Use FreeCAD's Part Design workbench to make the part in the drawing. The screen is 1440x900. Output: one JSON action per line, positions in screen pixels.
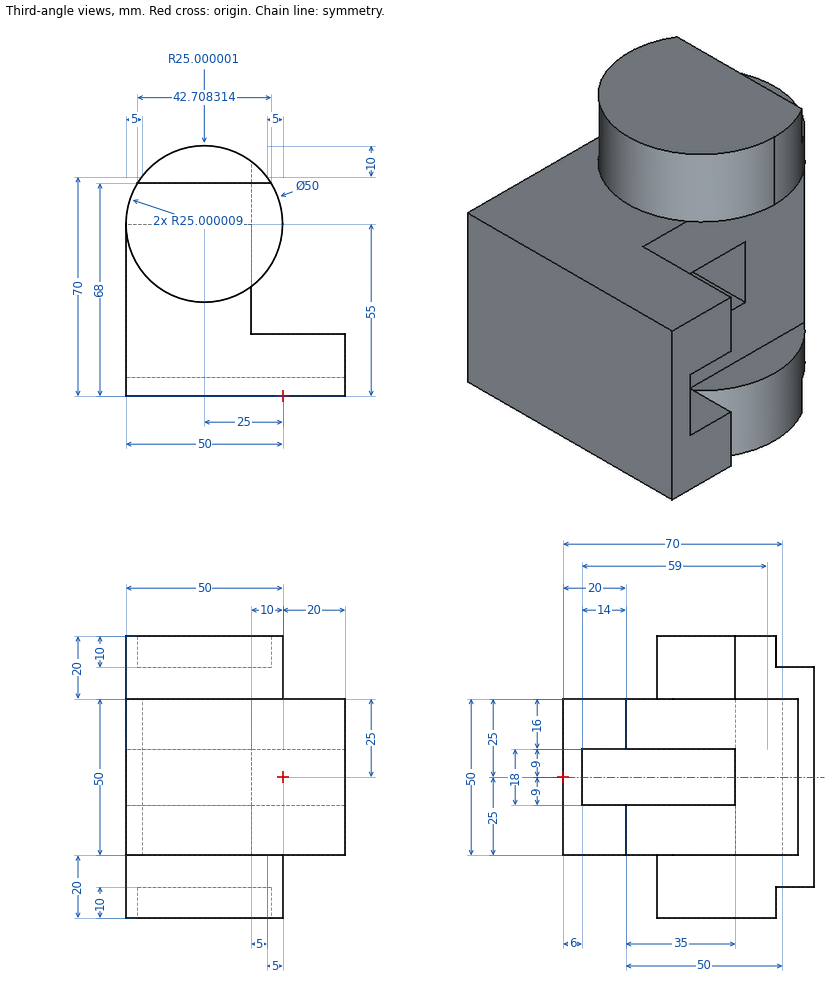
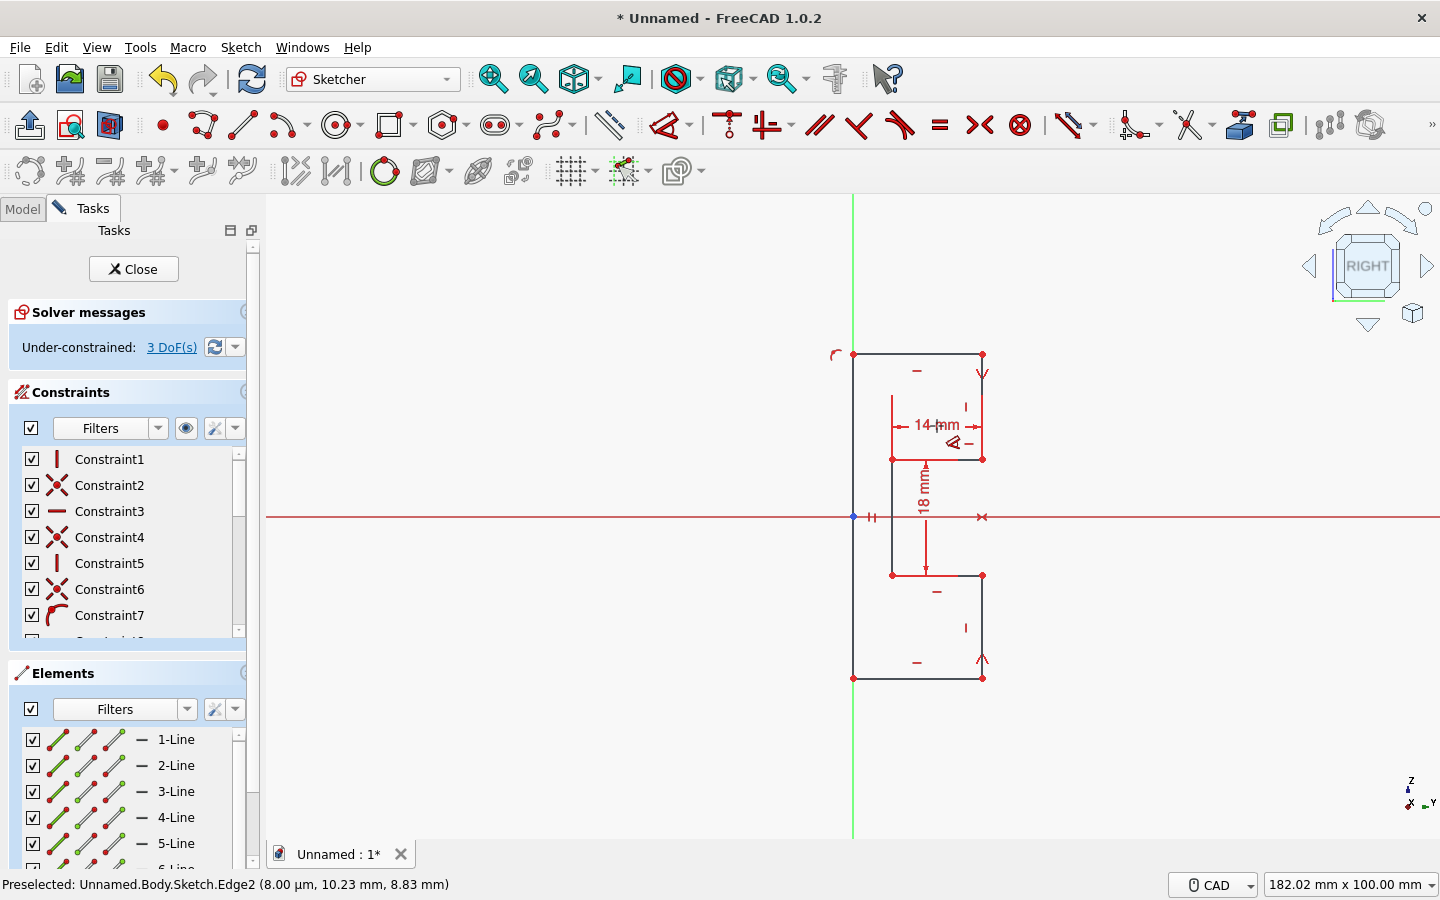
{"action": "left_click", "coordinate": [982, 428]}
{"action": "left_click", "coordinate": [1016, 407]}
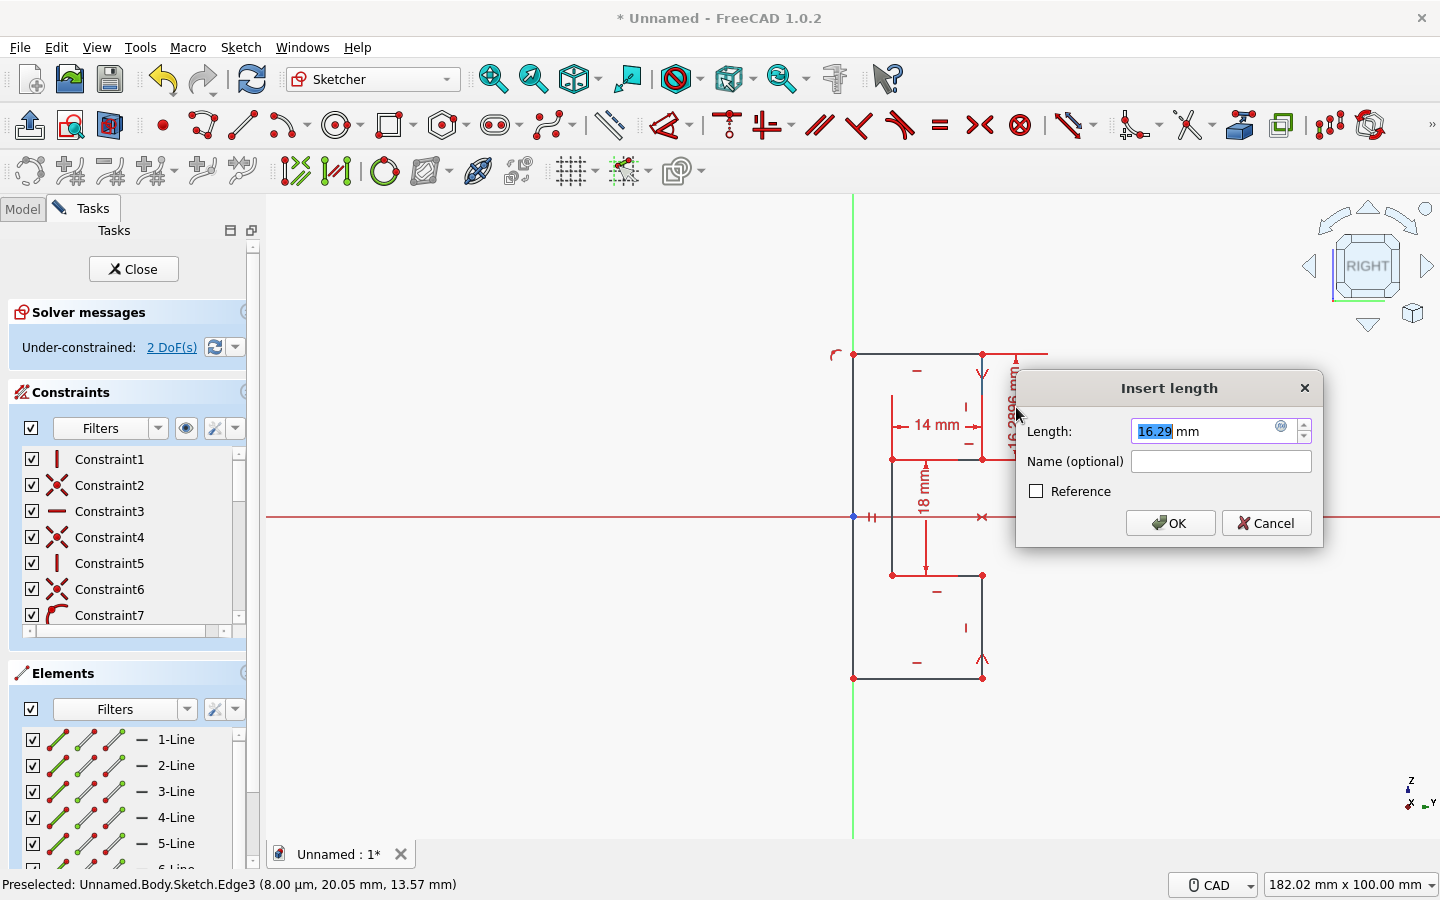
{"action": "type", "text": "16"}
{"action": "key", "text": "Return"}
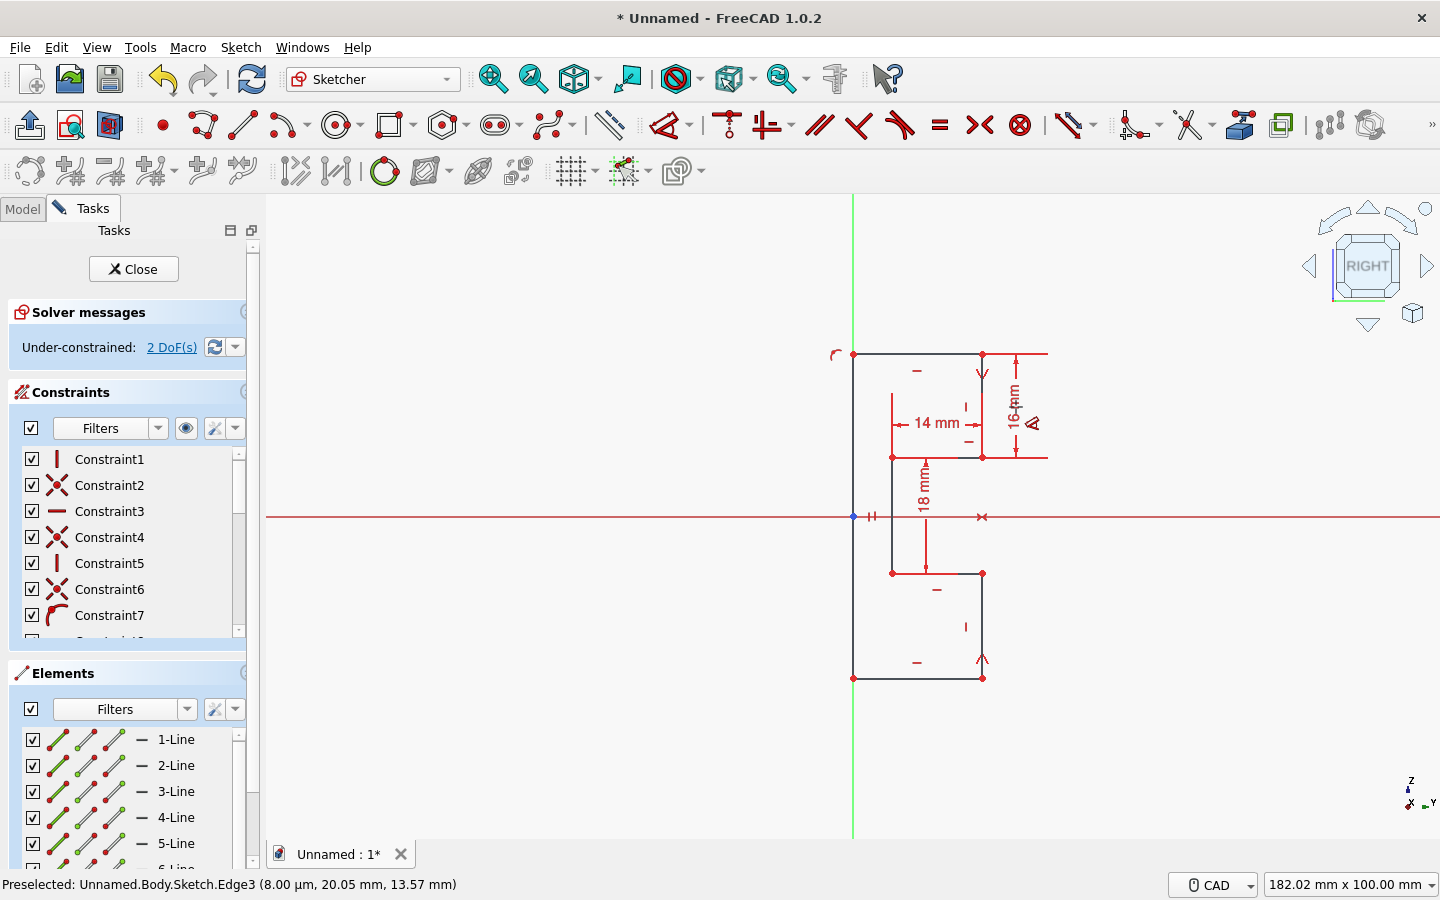
{"action": "left_click", "coordinate": [944, 354]}
{"action": "left_click", "coordinate": [918, 320]}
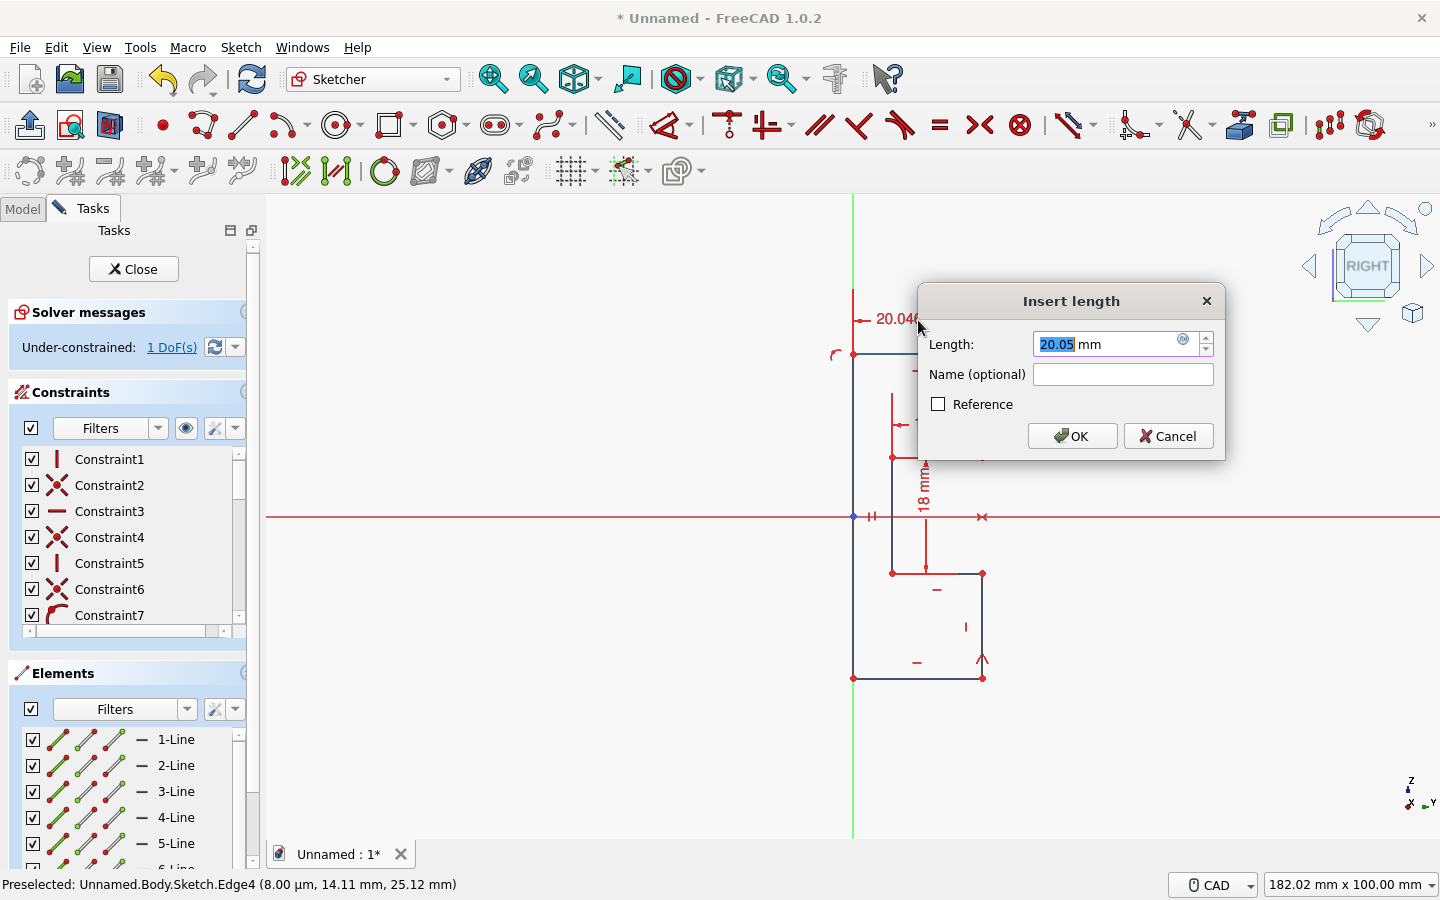
{"action": "type", "text": "20"}
{"action": "key", "text": "Return"}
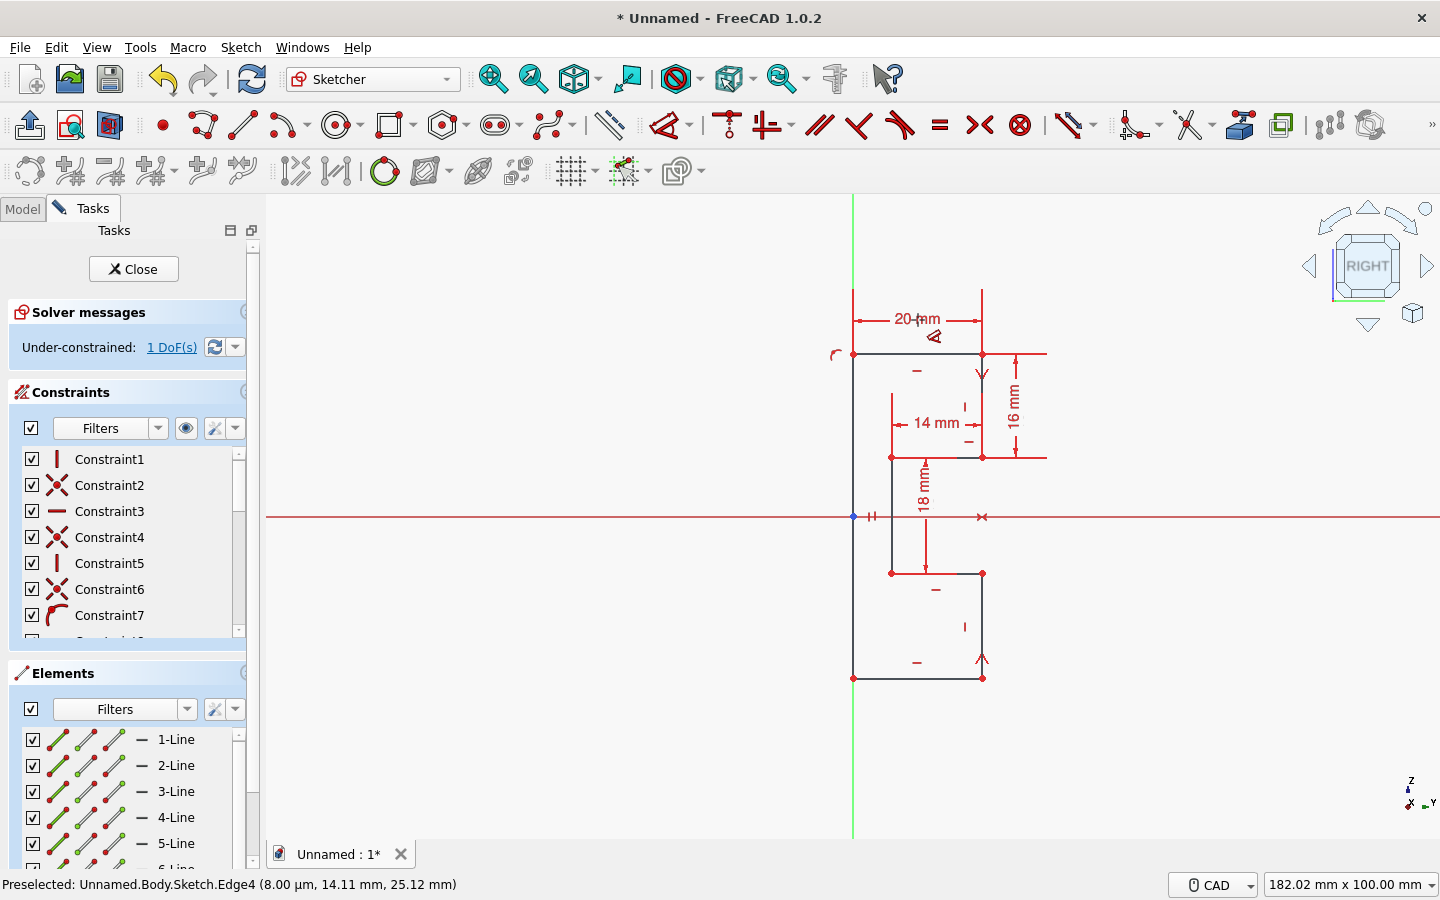
{"action": "left_click", "coordinate": [853, 452]}
{"action": "left_click", "coordinate": [819, 442]}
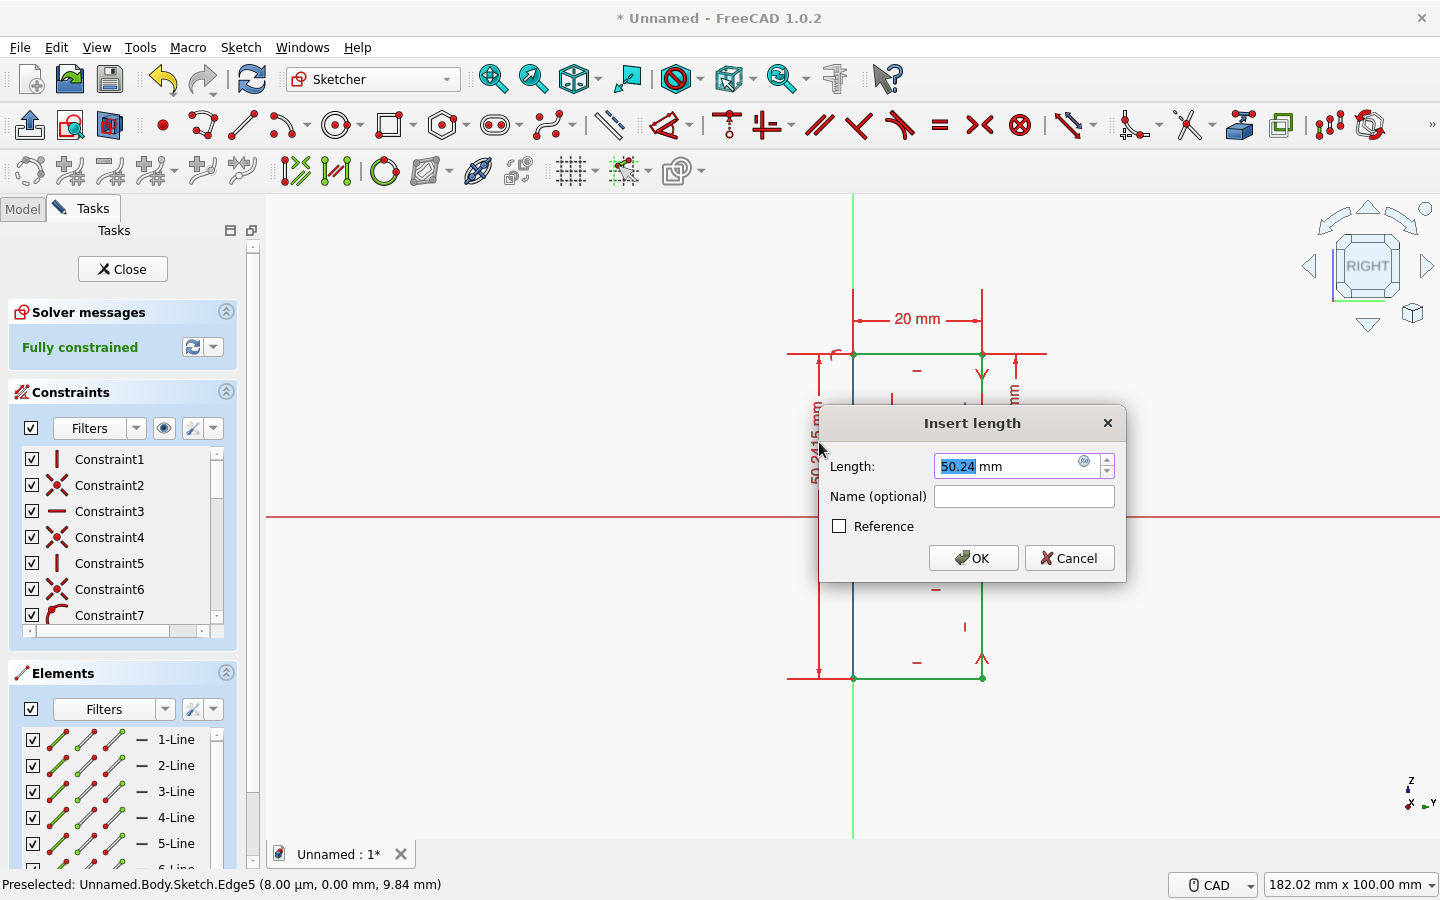
{"action": "type", "text": "50"}
{"action": "key", "text": "Return"}
{"action": "key", "text": "Escape"}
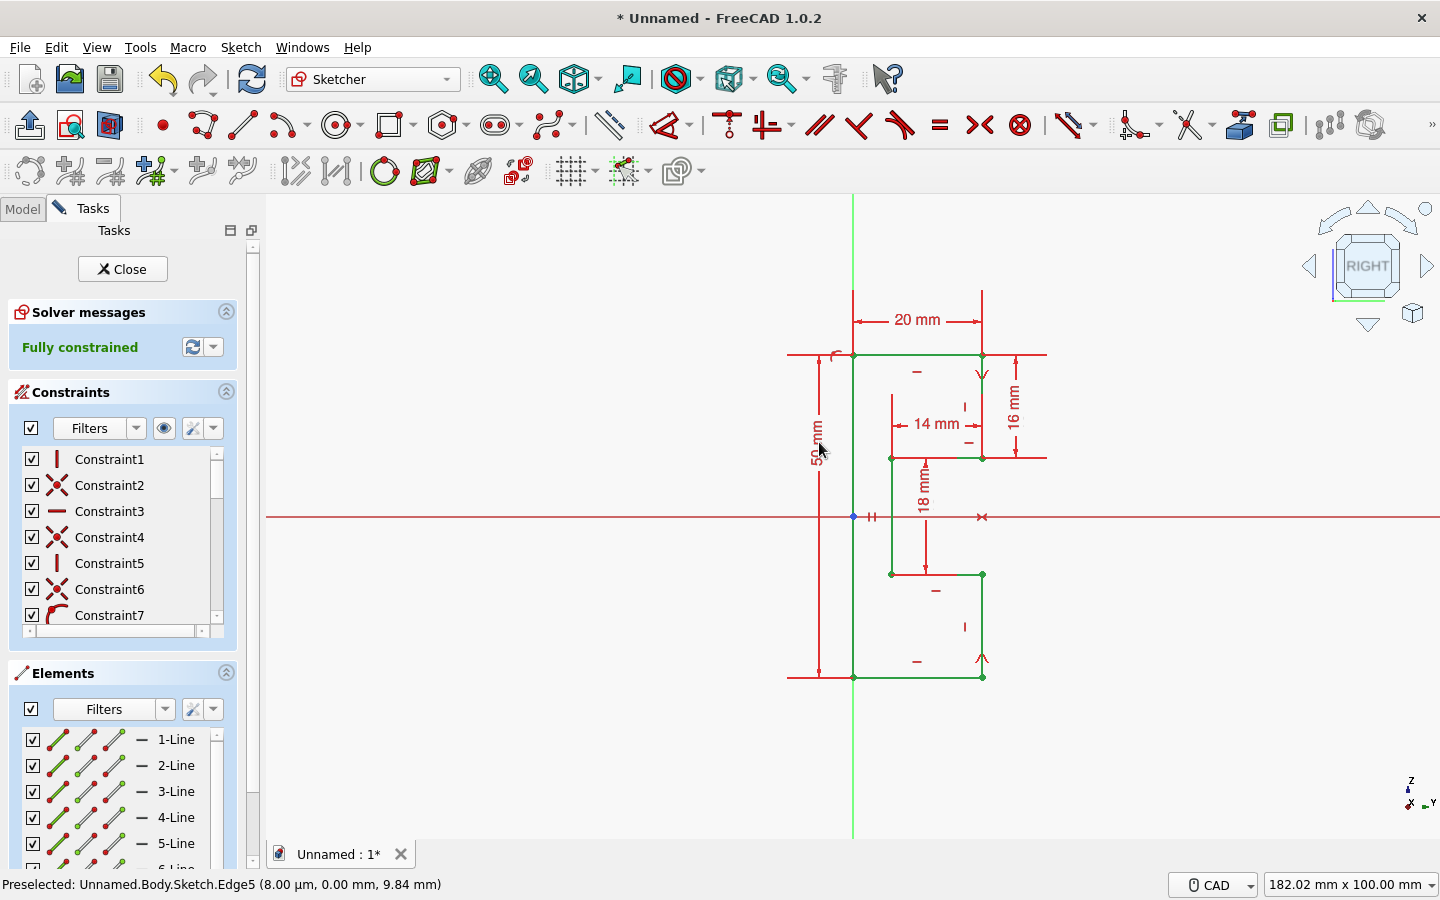
{"action": "left_click", "coordinate": [123, 269]}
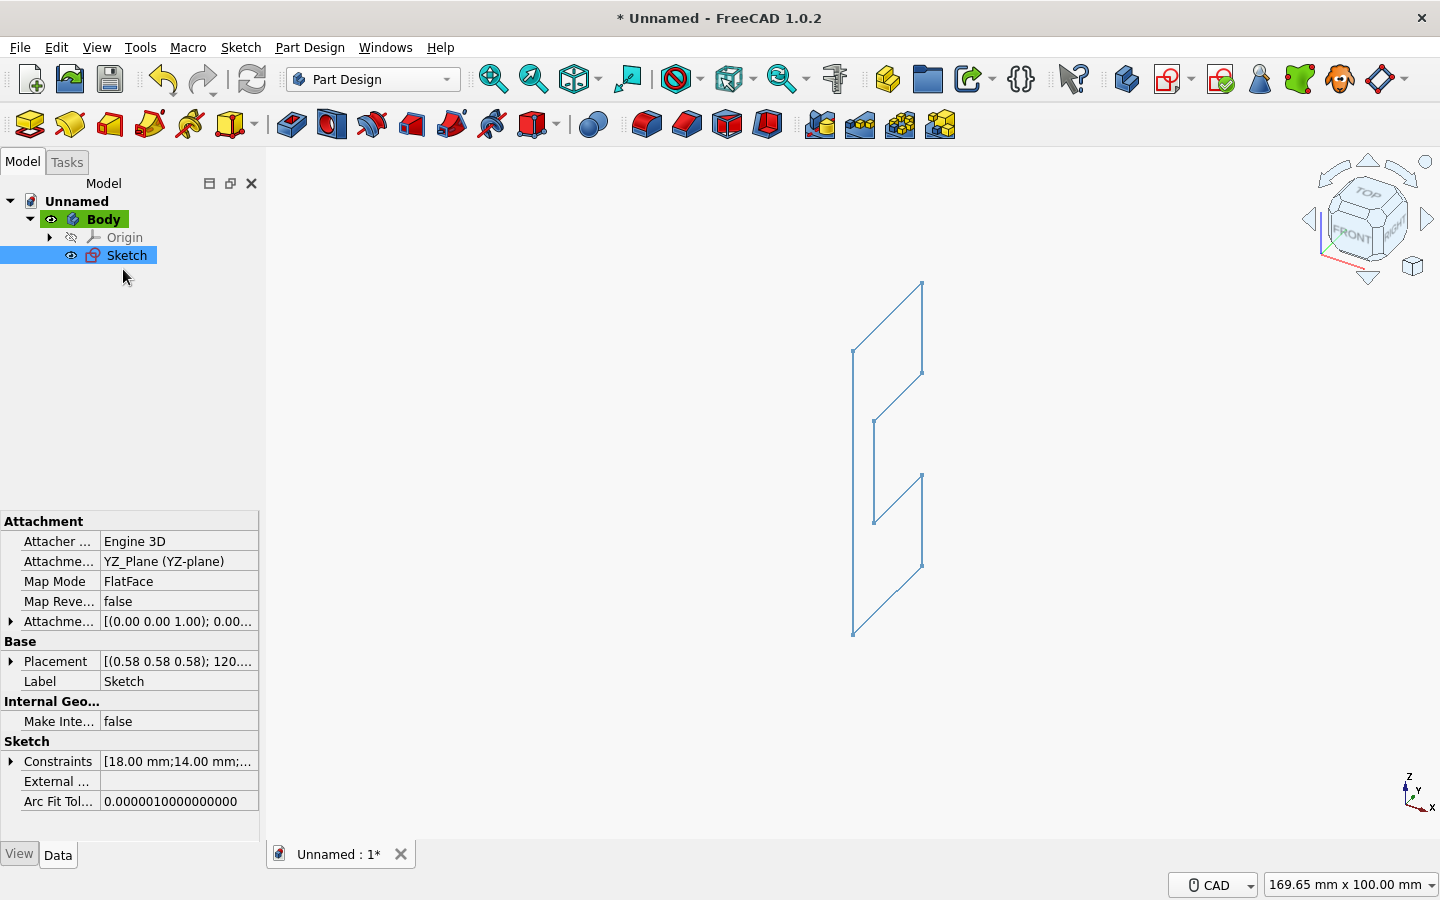
{"action": "left_click", "coordinate": [30, 124]}